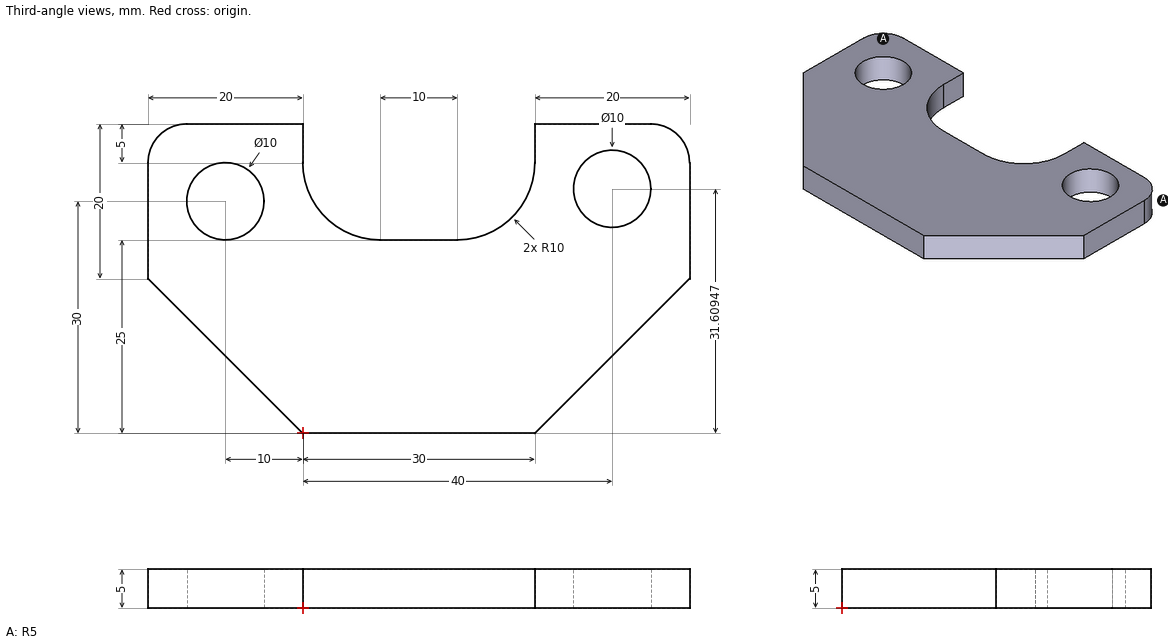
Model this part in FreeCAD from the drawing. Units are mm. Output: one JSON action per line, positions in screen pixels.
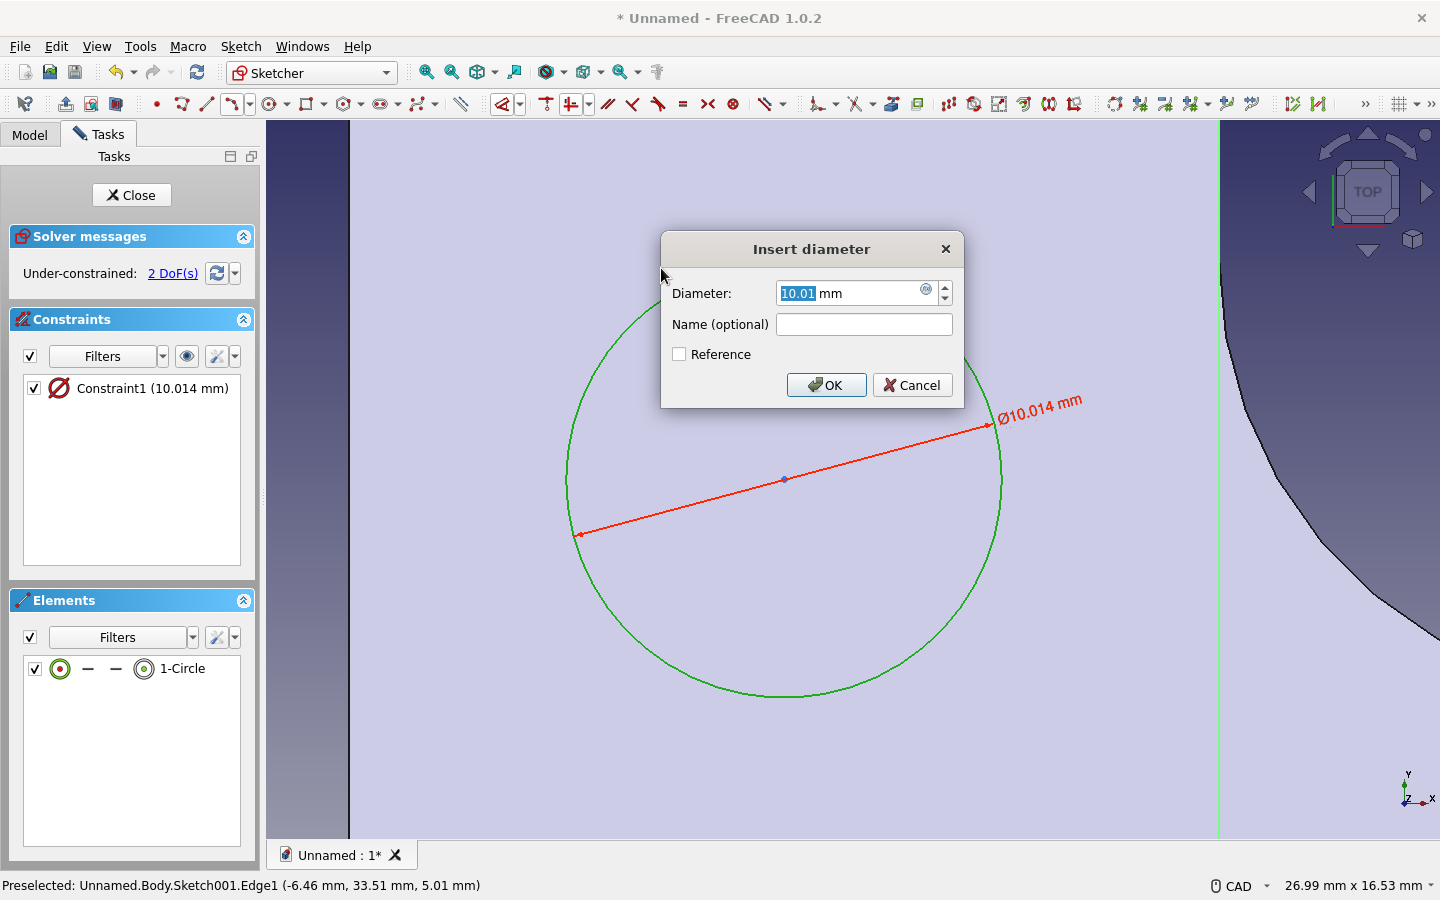
{"action": "type", "text": "10"}
{"action": "key", "text": "Return"}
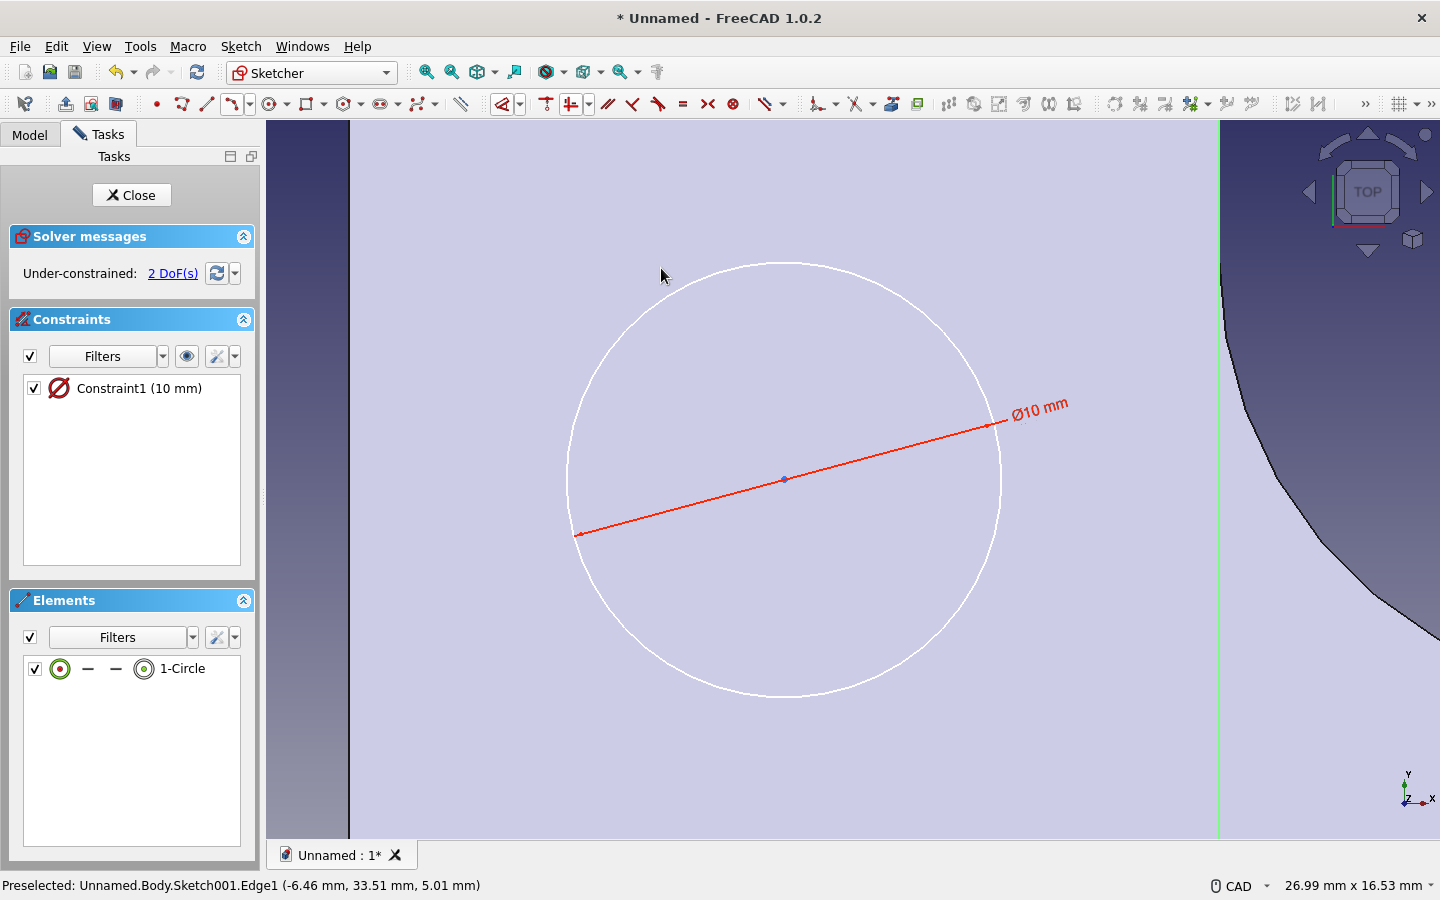
{"action": "left_click", "coordinate": [784, 480]}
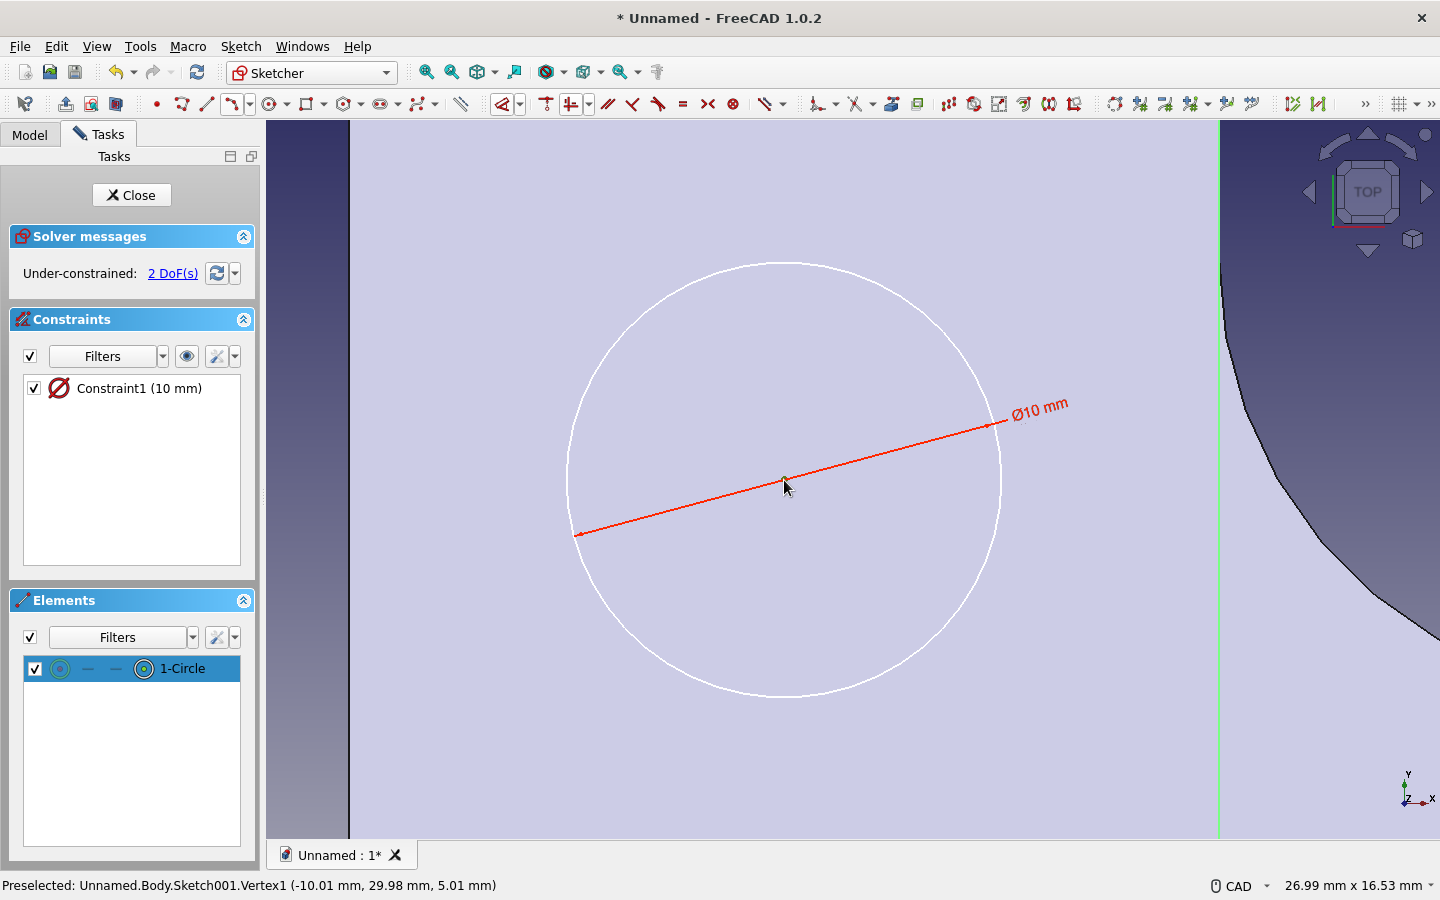
{"action": "left_click", "coordinate": [520, 104]}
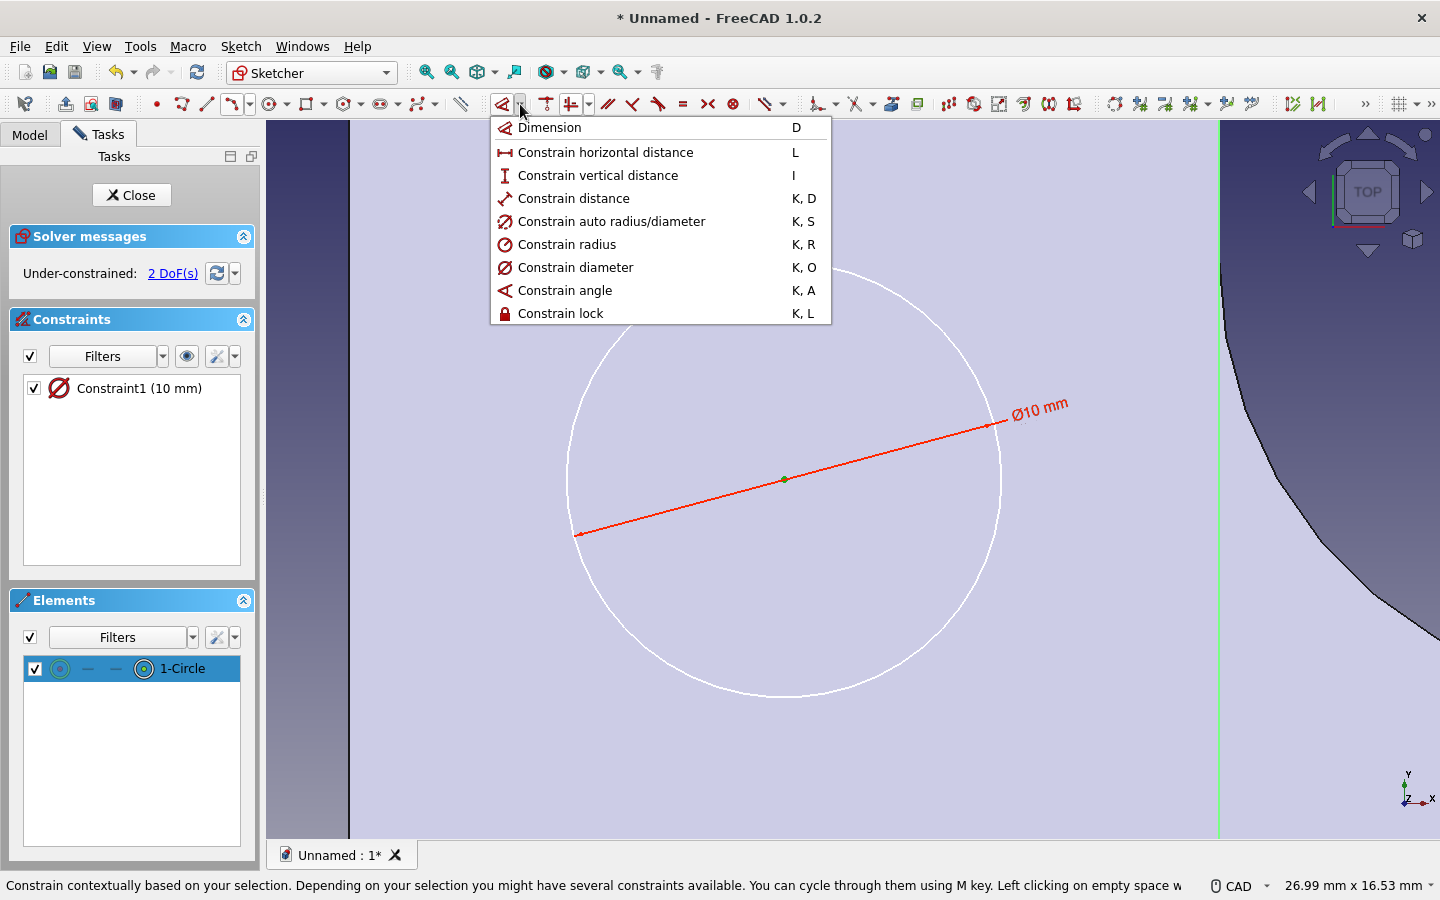
{"action": "left_click", "coordinate": [661, 152]}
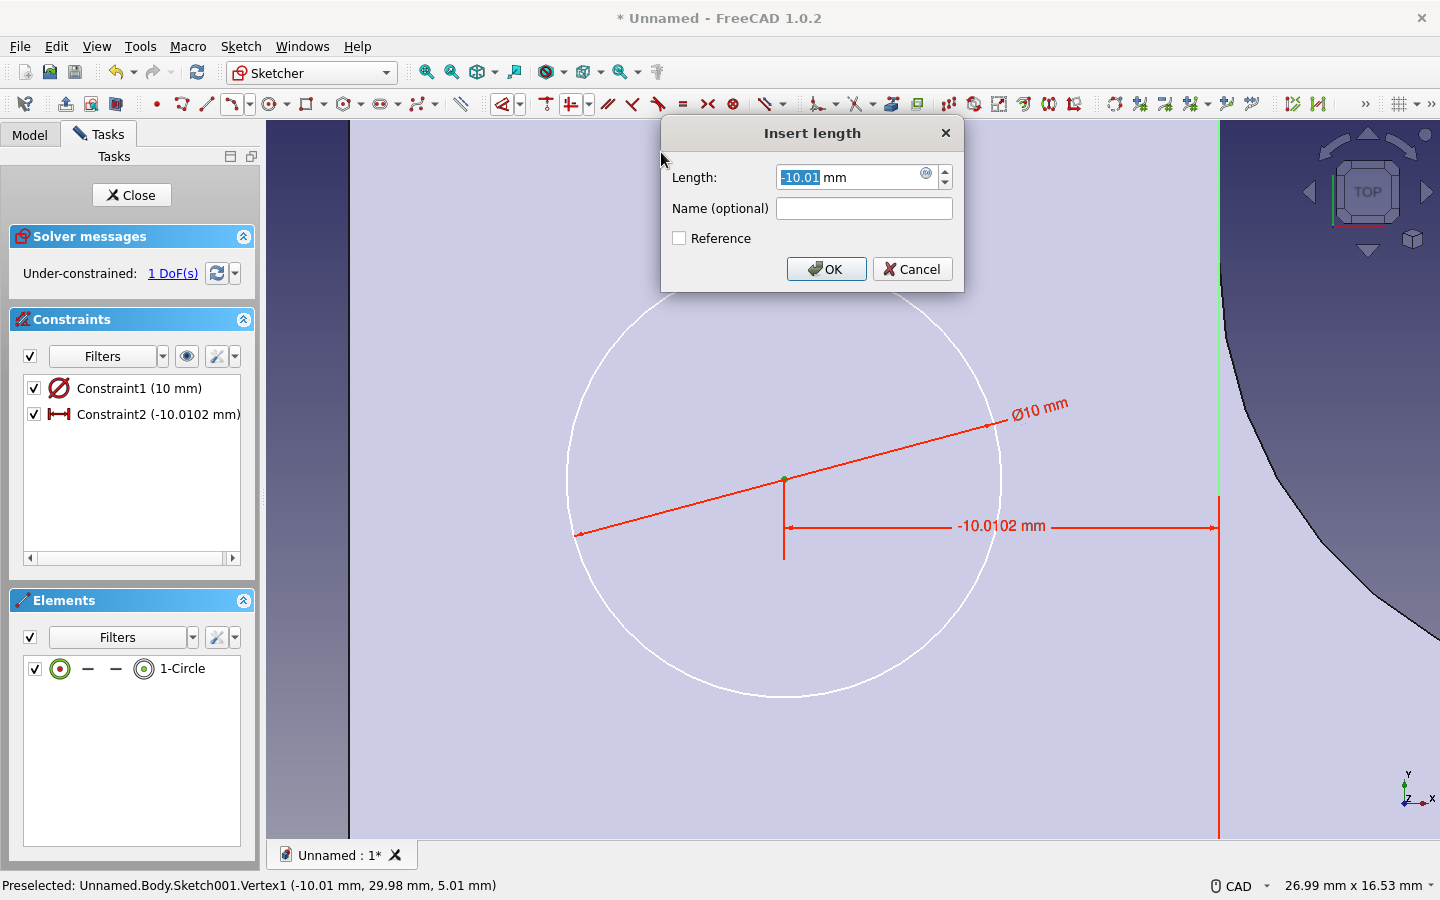
{"action": "type", "text": "-10"}
{"action": "key", "text": "Return"}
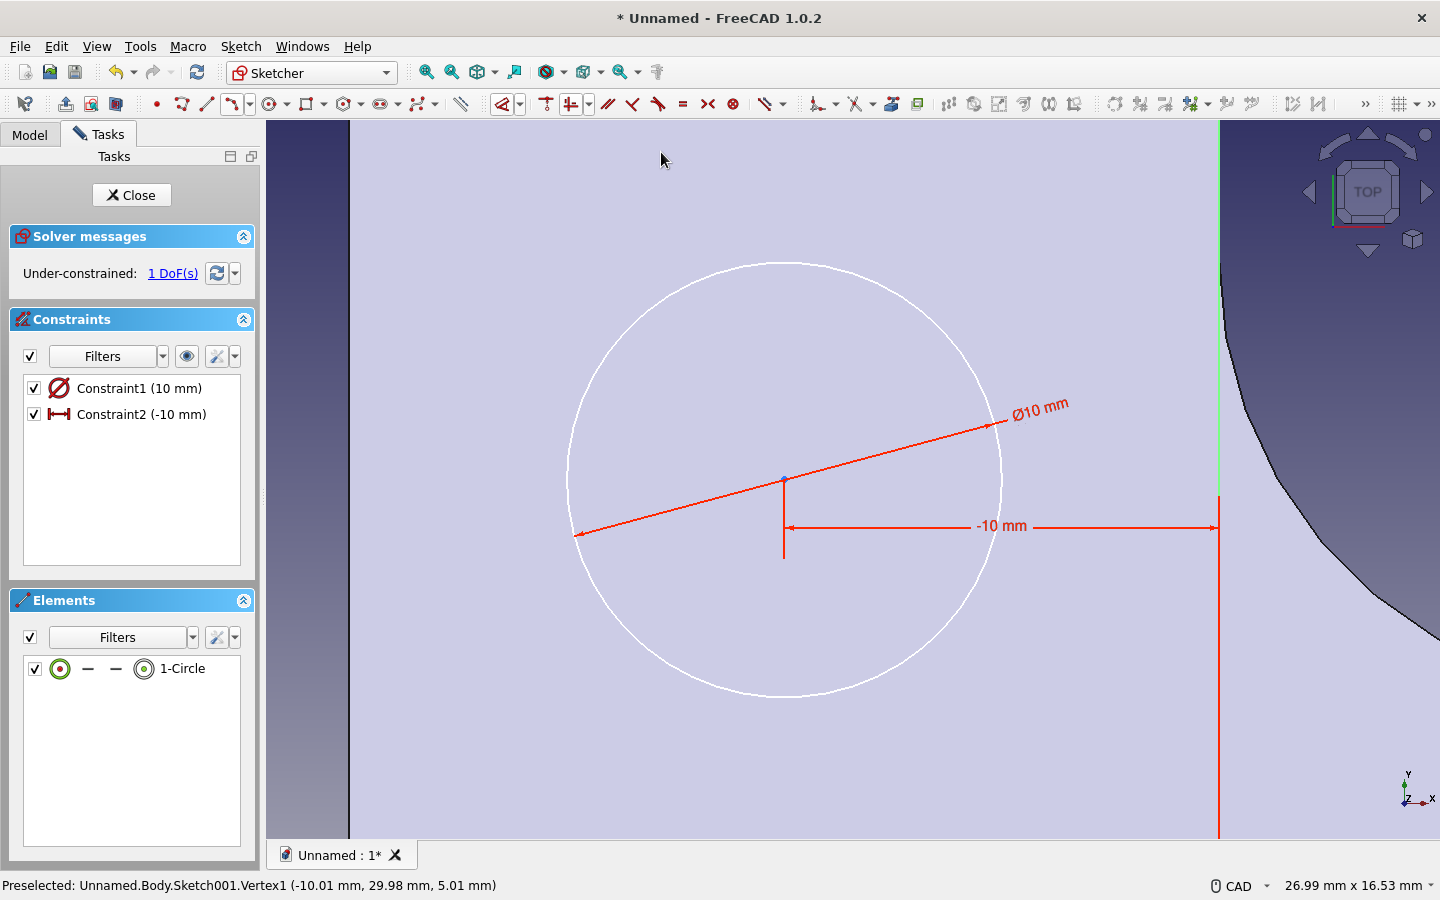
{"action": "left_click", "coordinate": [784, 480]}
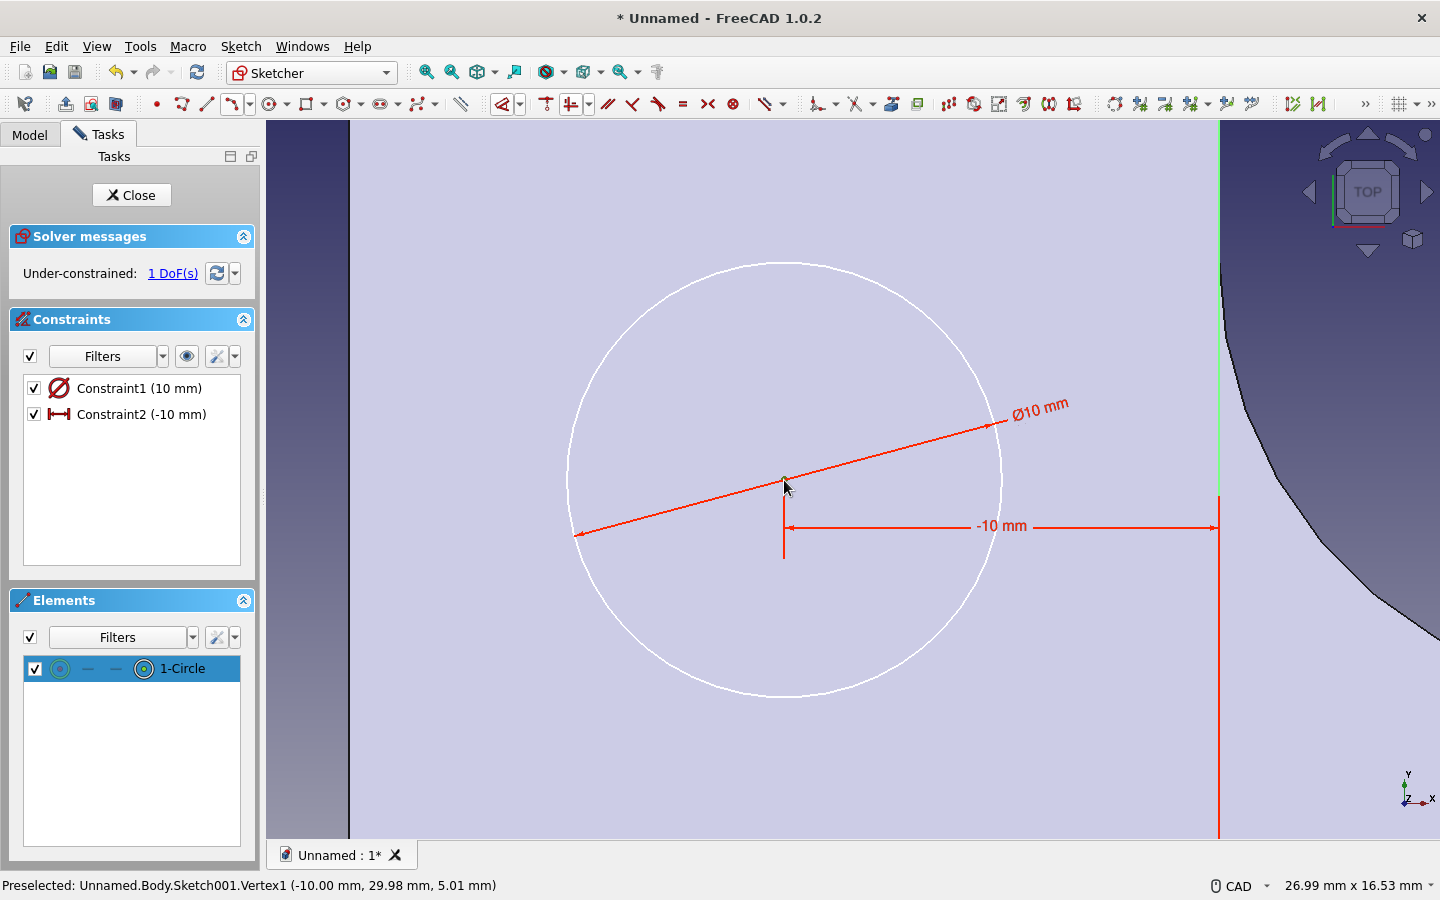
{"action": "key", "text": "i"}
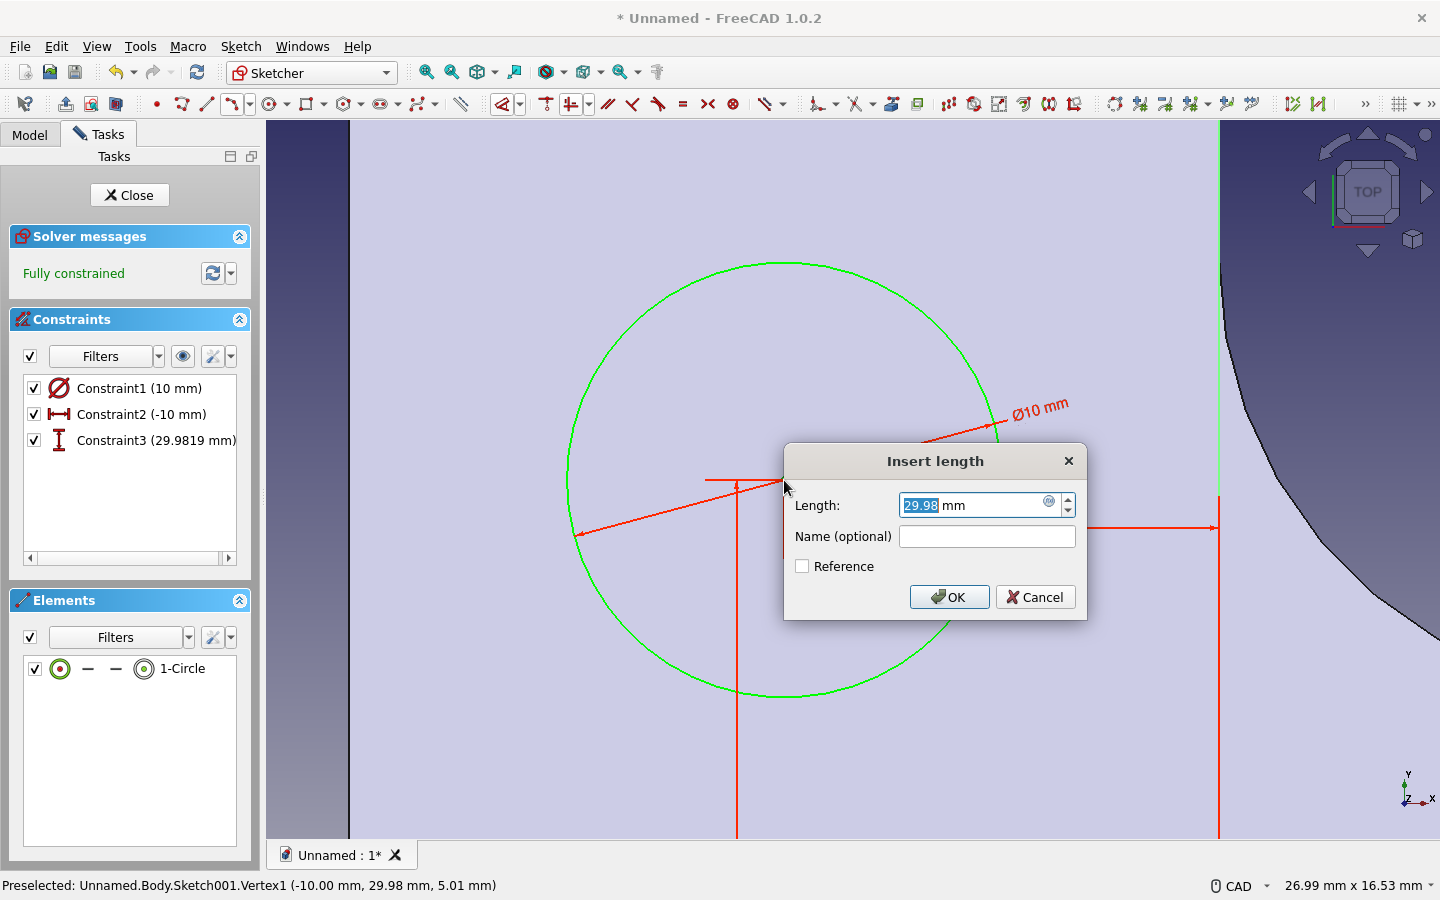
{"action": "type", "text": "30"}
{"action": "key", "text": "Return"}